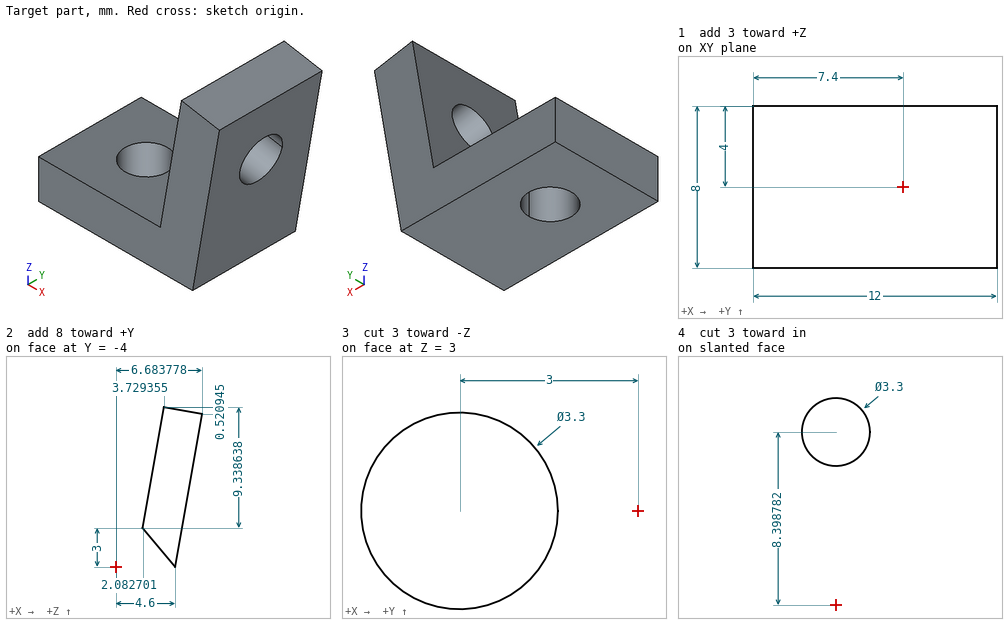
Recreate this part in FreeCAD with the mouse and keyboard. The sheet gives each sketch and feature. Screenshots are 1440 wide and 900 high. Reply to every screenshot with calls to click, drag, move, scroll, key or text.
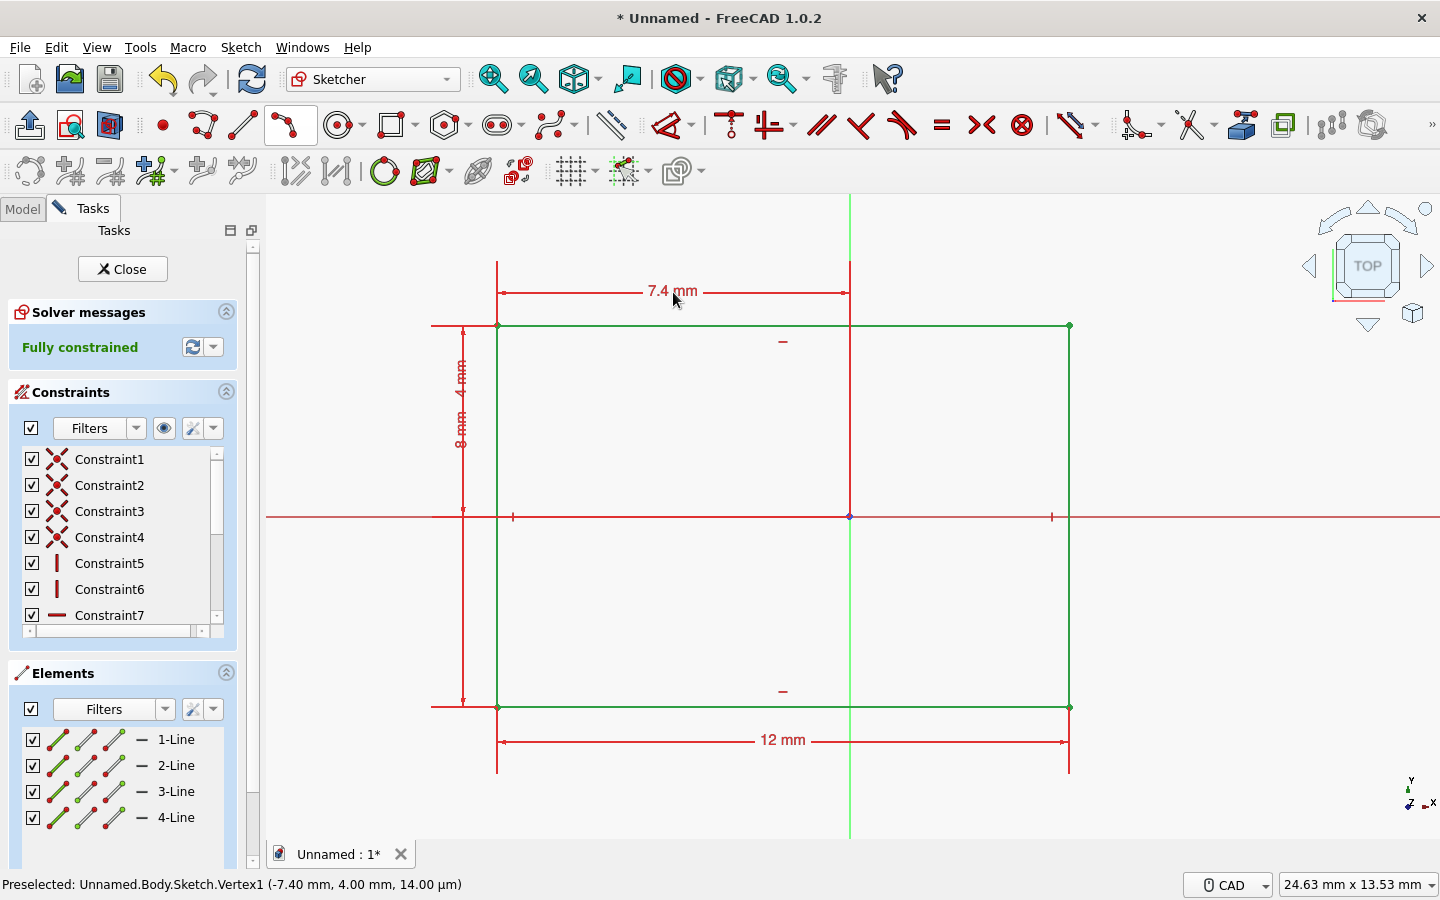
click(123, 269)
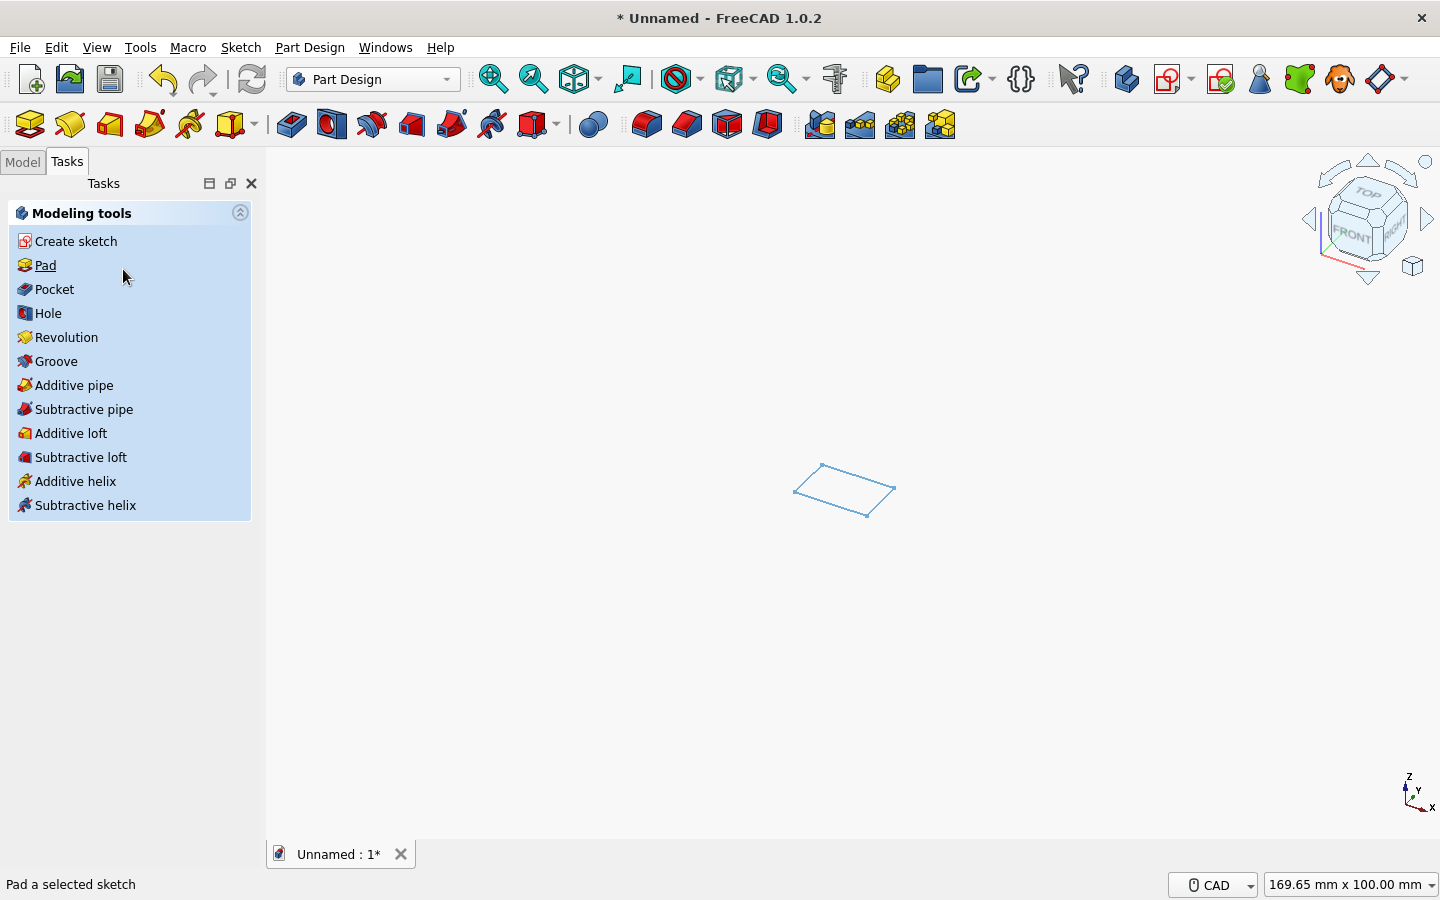
click(30, 124)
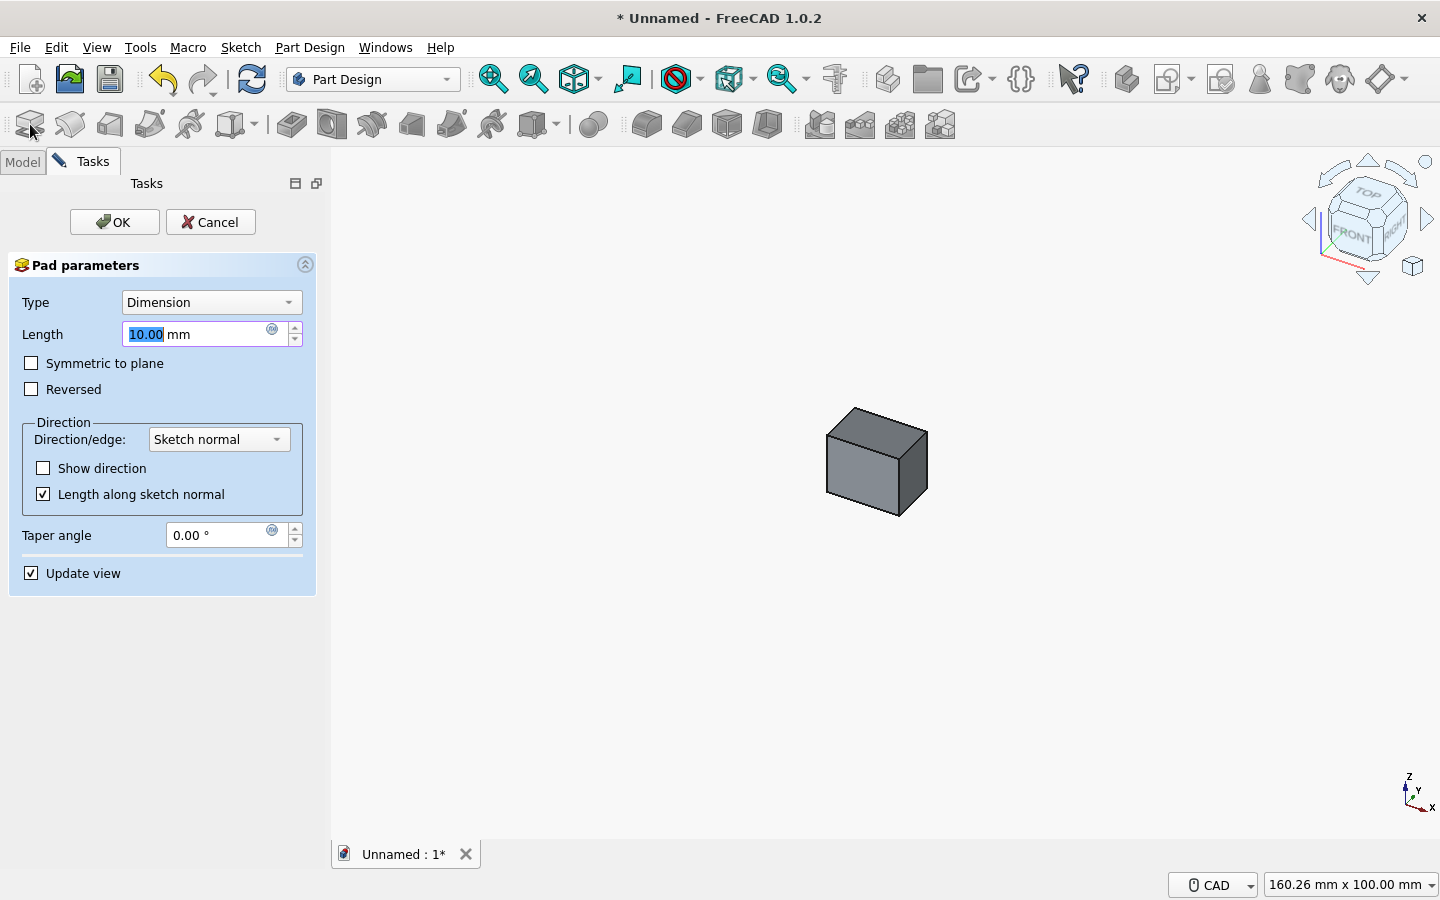
text(3)
key(Tab)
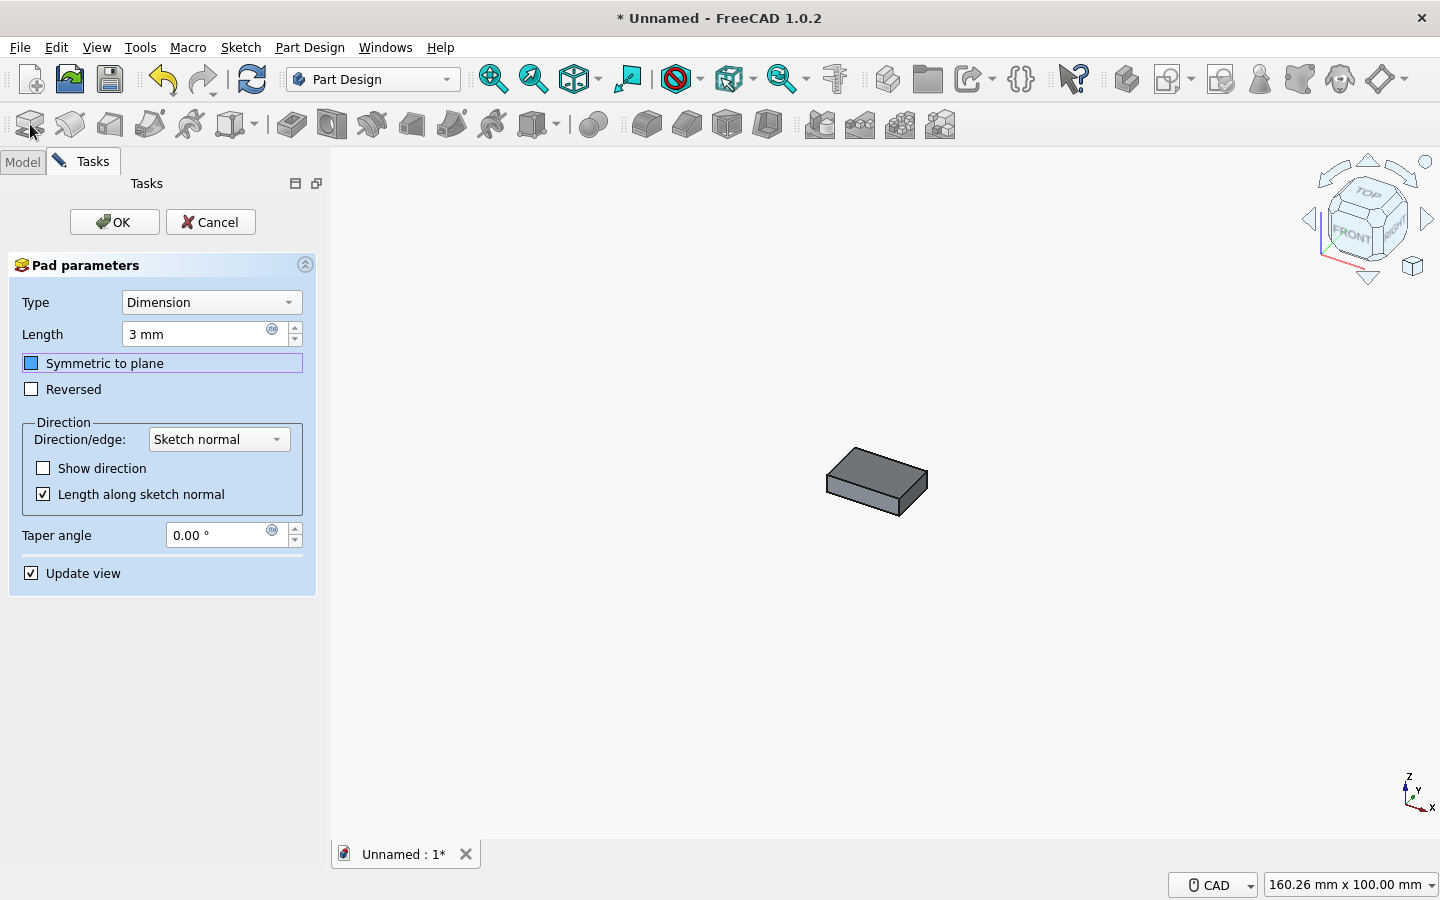
click(115, 222)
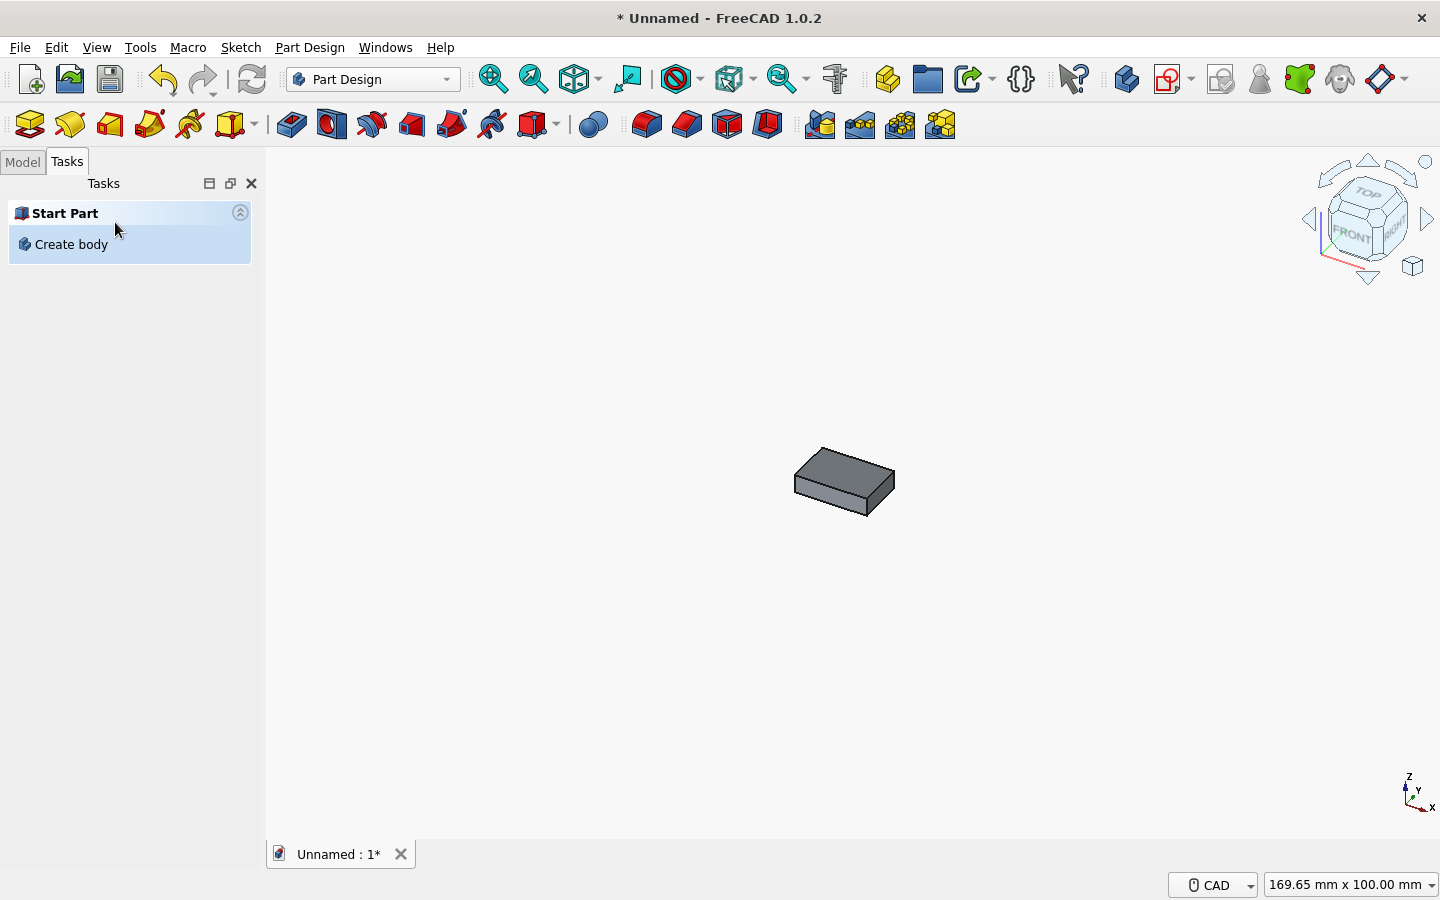
click(494, 80)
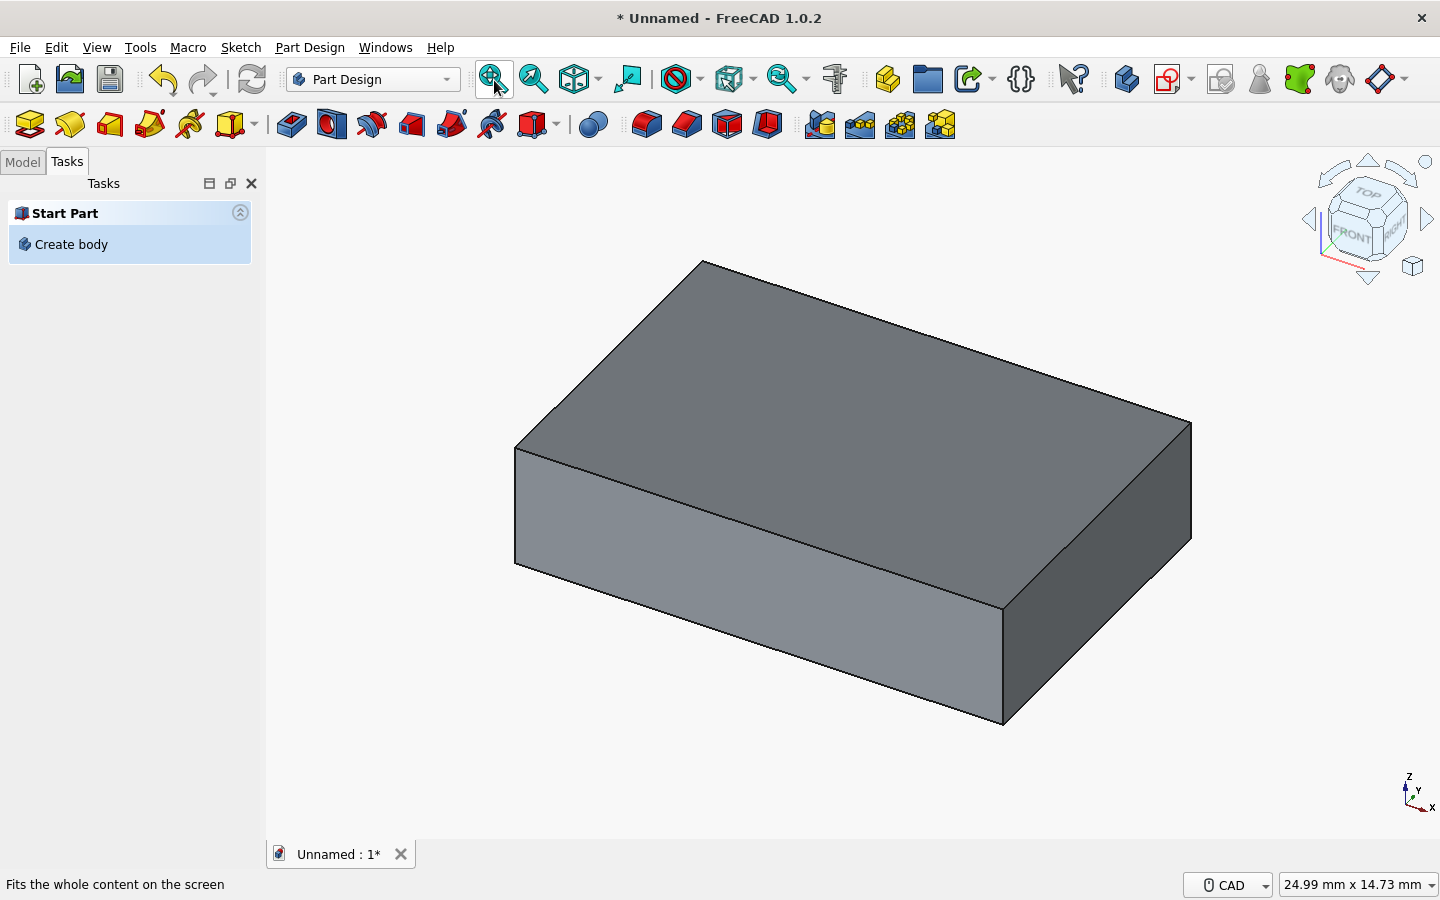
click(899, 632)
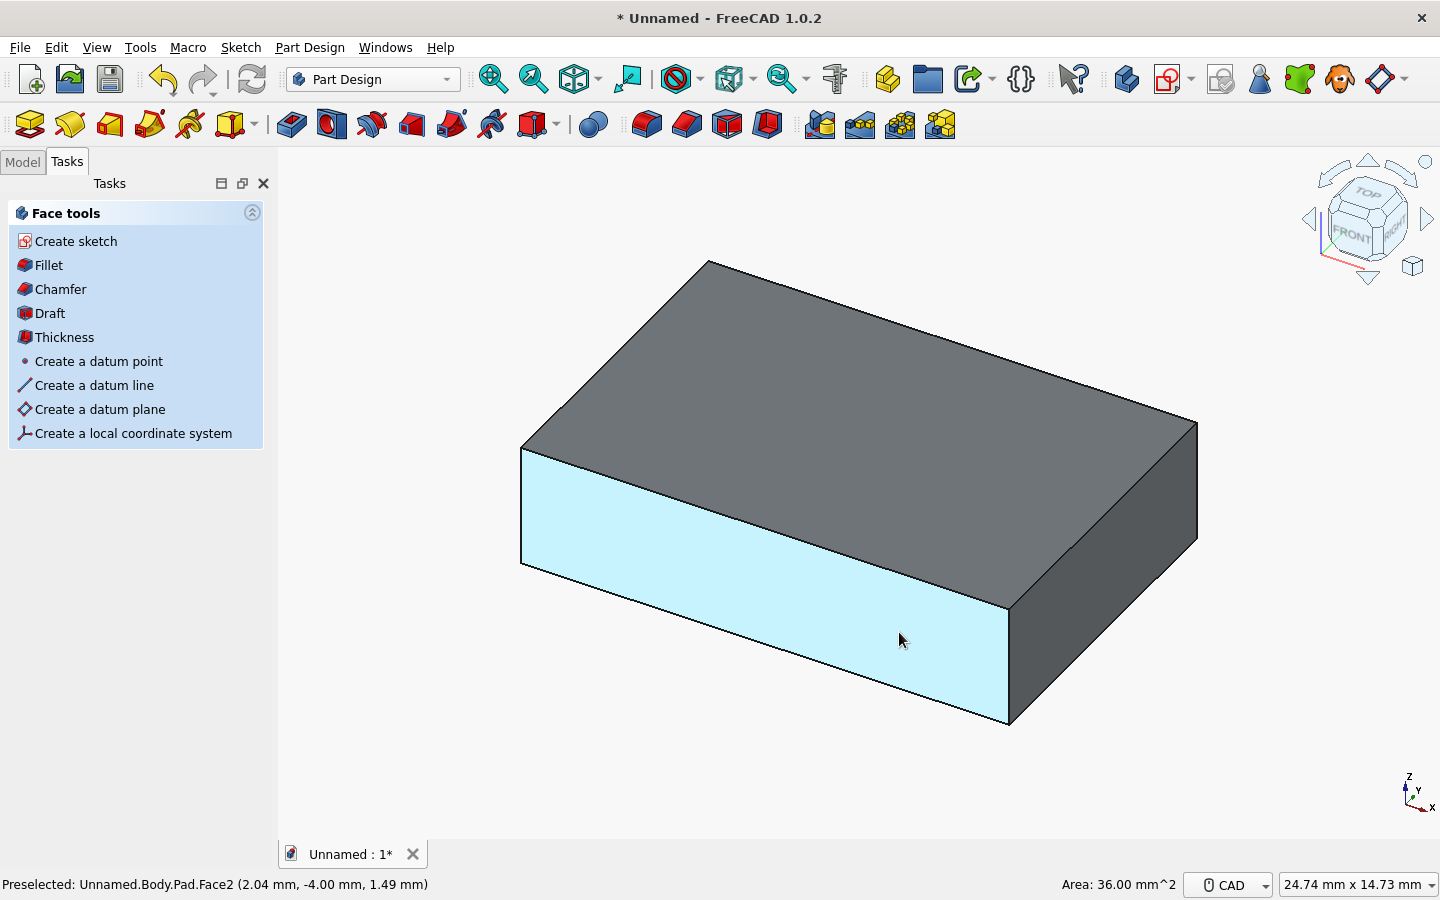
click(1168, 80)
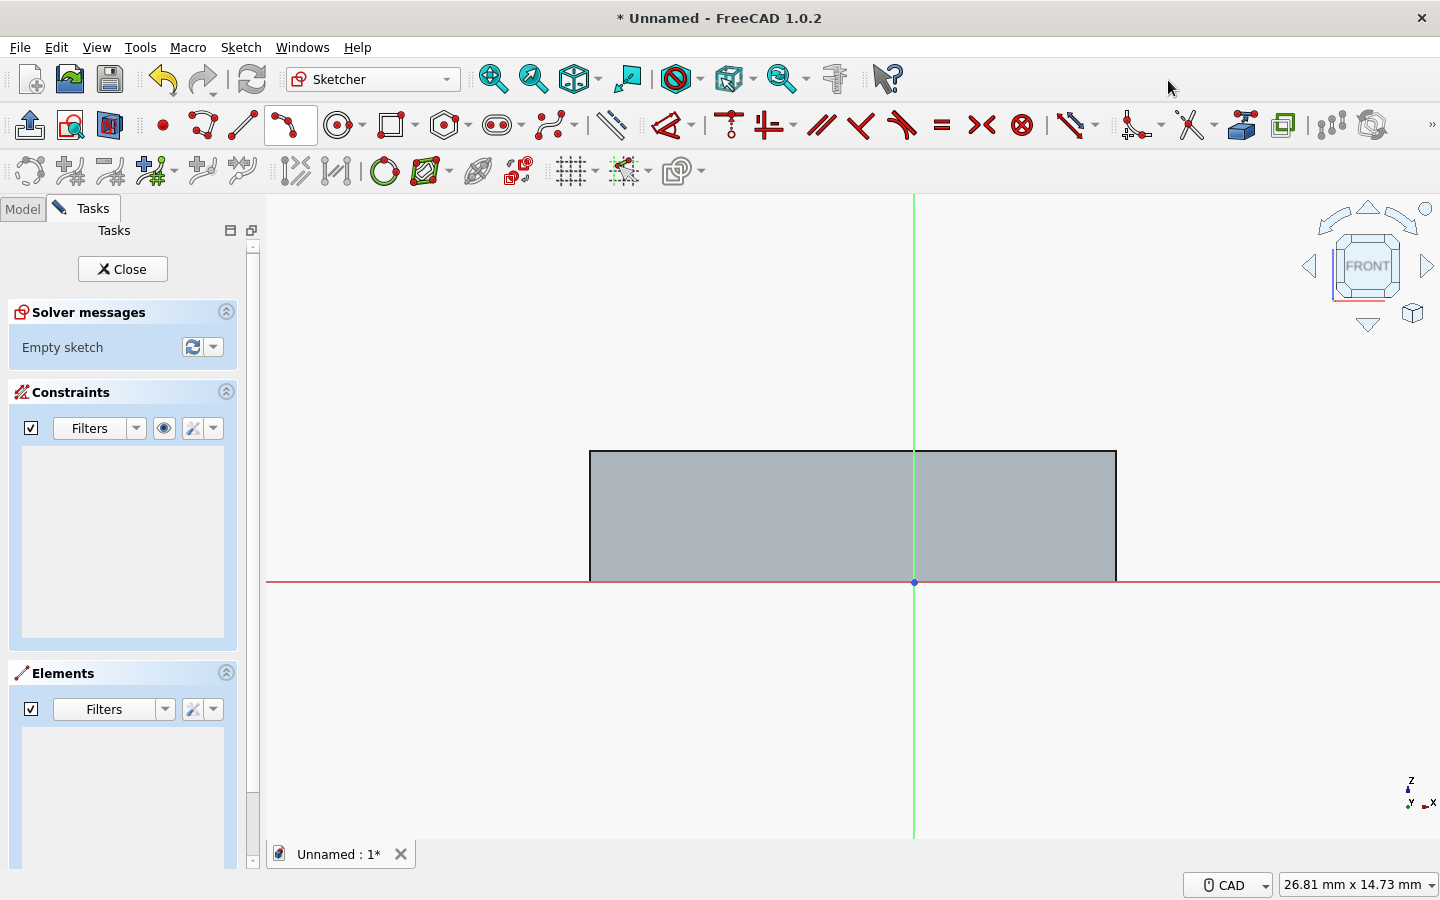
scroll(294, 811, down, 2)